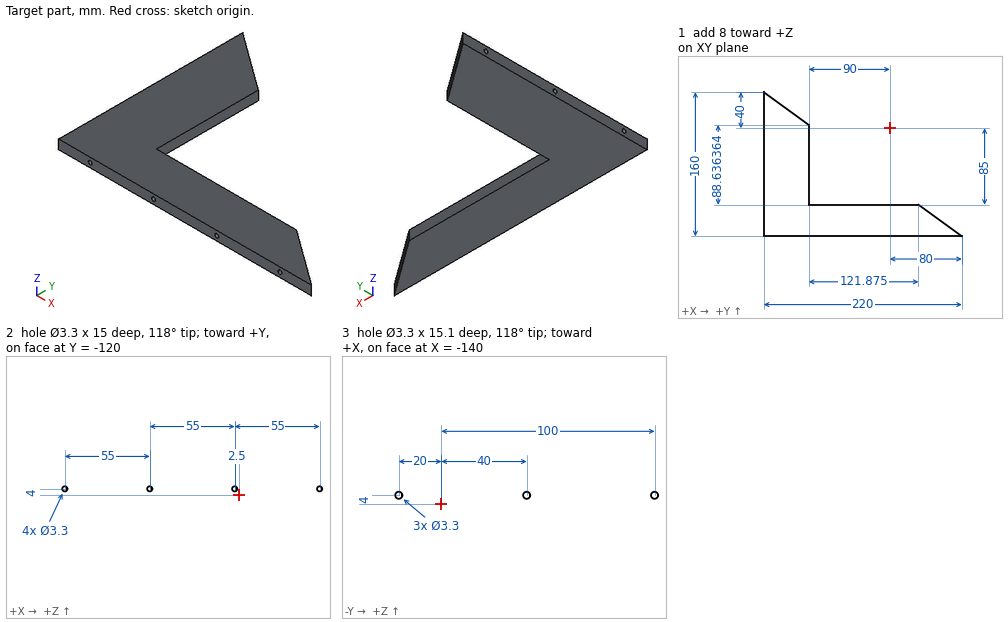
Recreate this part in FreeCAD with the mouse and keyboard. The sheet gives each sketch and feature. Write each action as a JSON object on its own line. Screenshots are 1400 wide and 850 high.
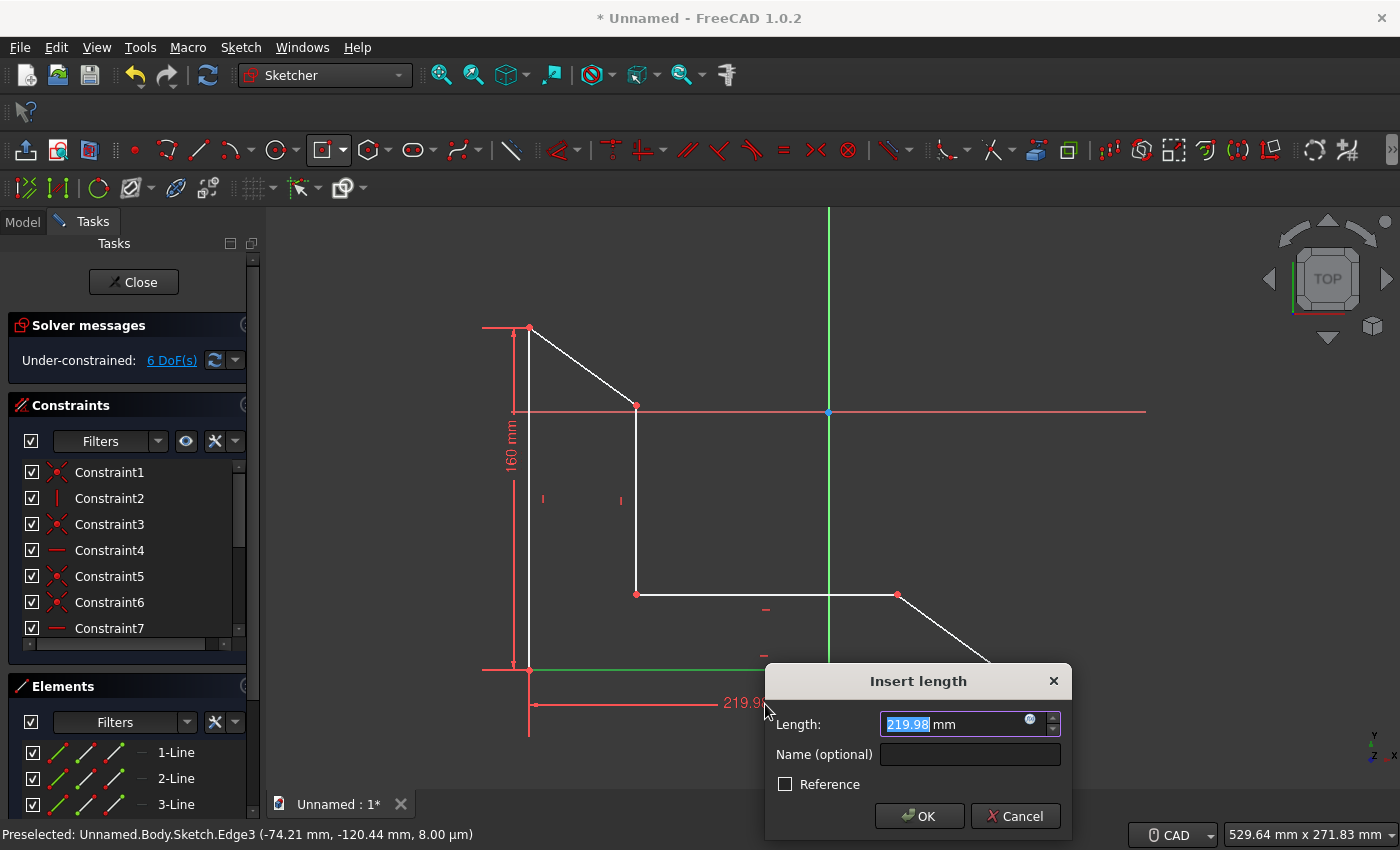
{"action": "type", "text": "220"}
{"action": "key", "text": "Return"}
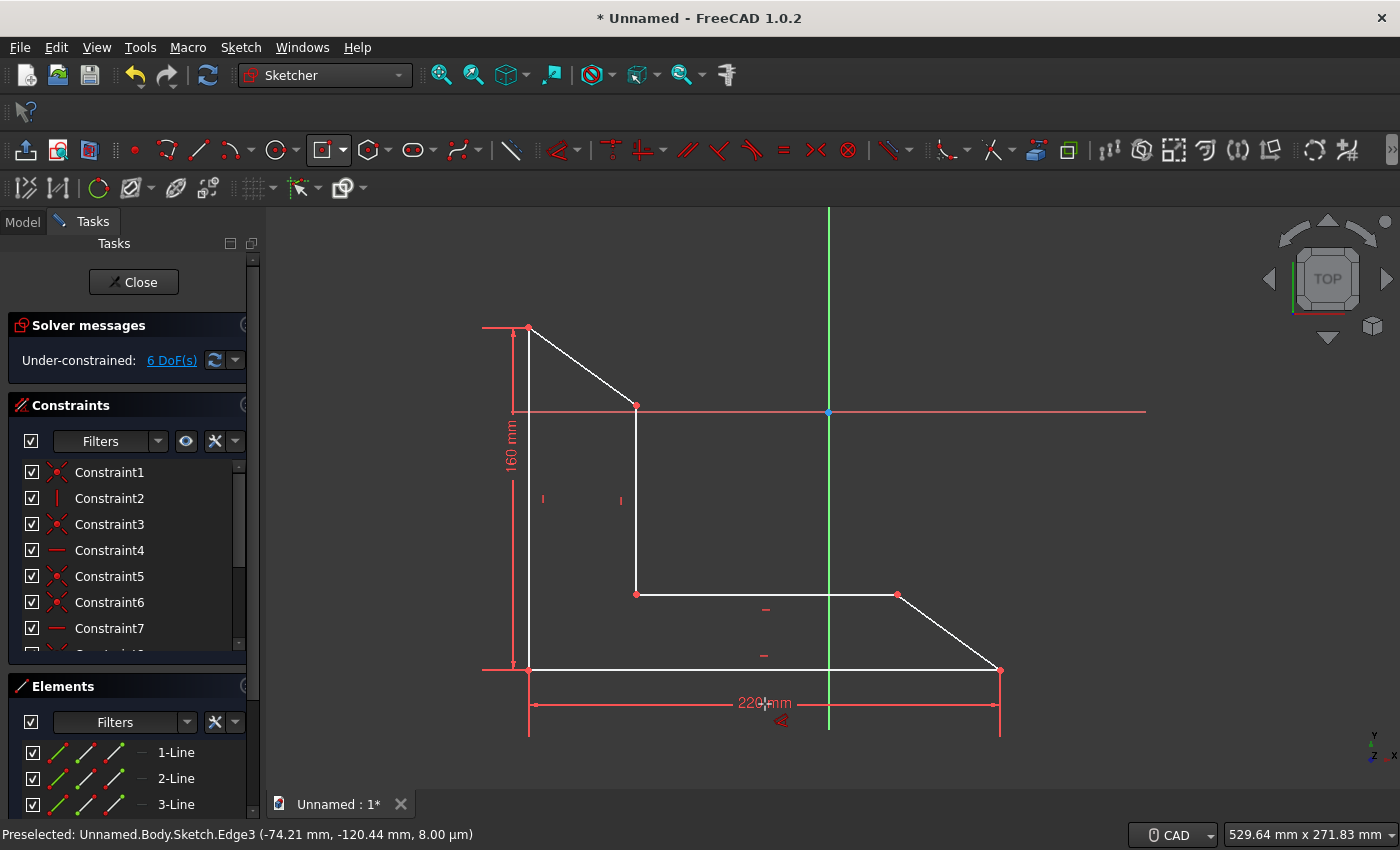
{"action": "left_click", "coordinate": [636, 405]}
{"action": "left_click", "coordinate": [732, 371]}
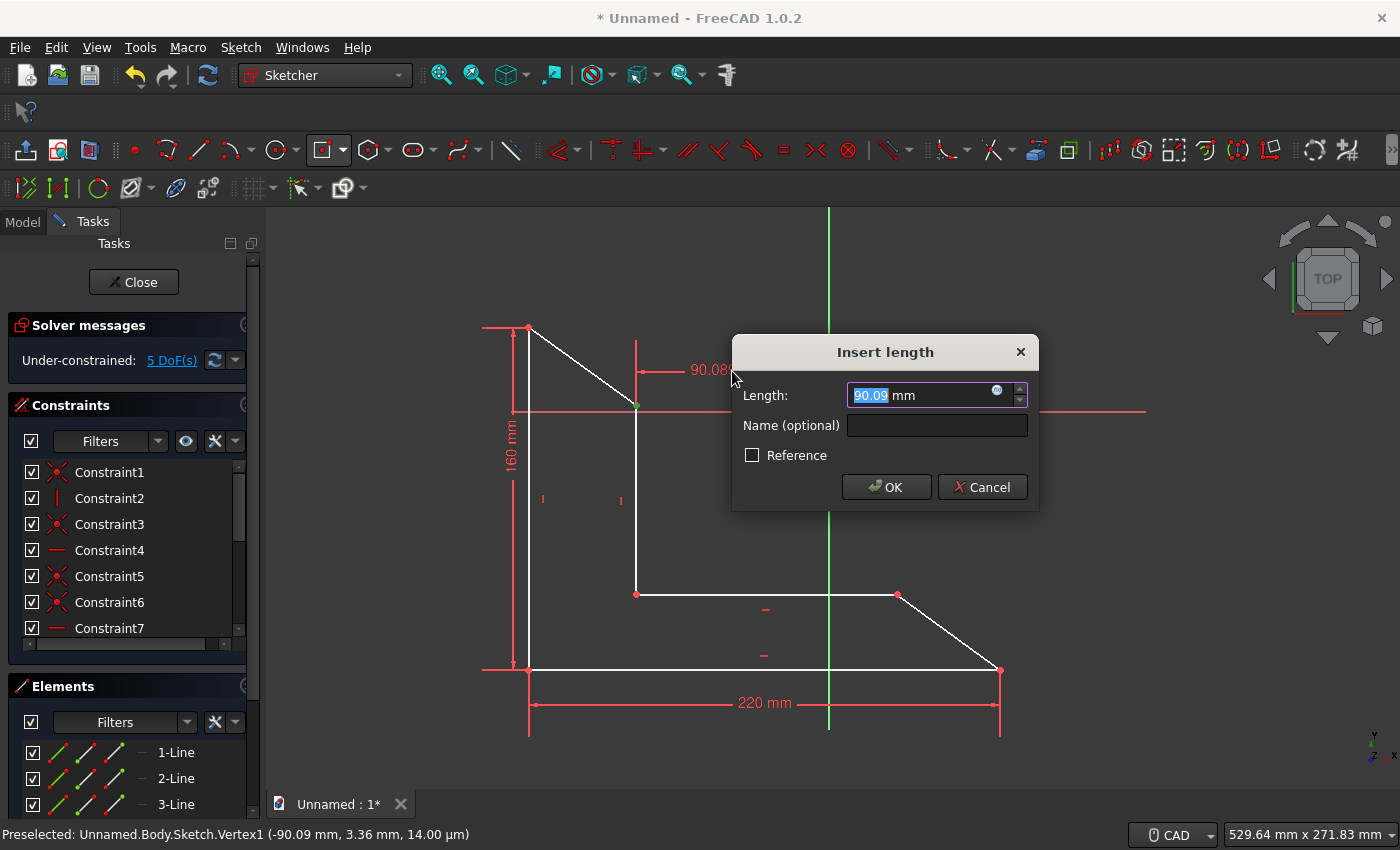
{"action": "type", "text": "90"}
{"action": "key", "text": "Return"}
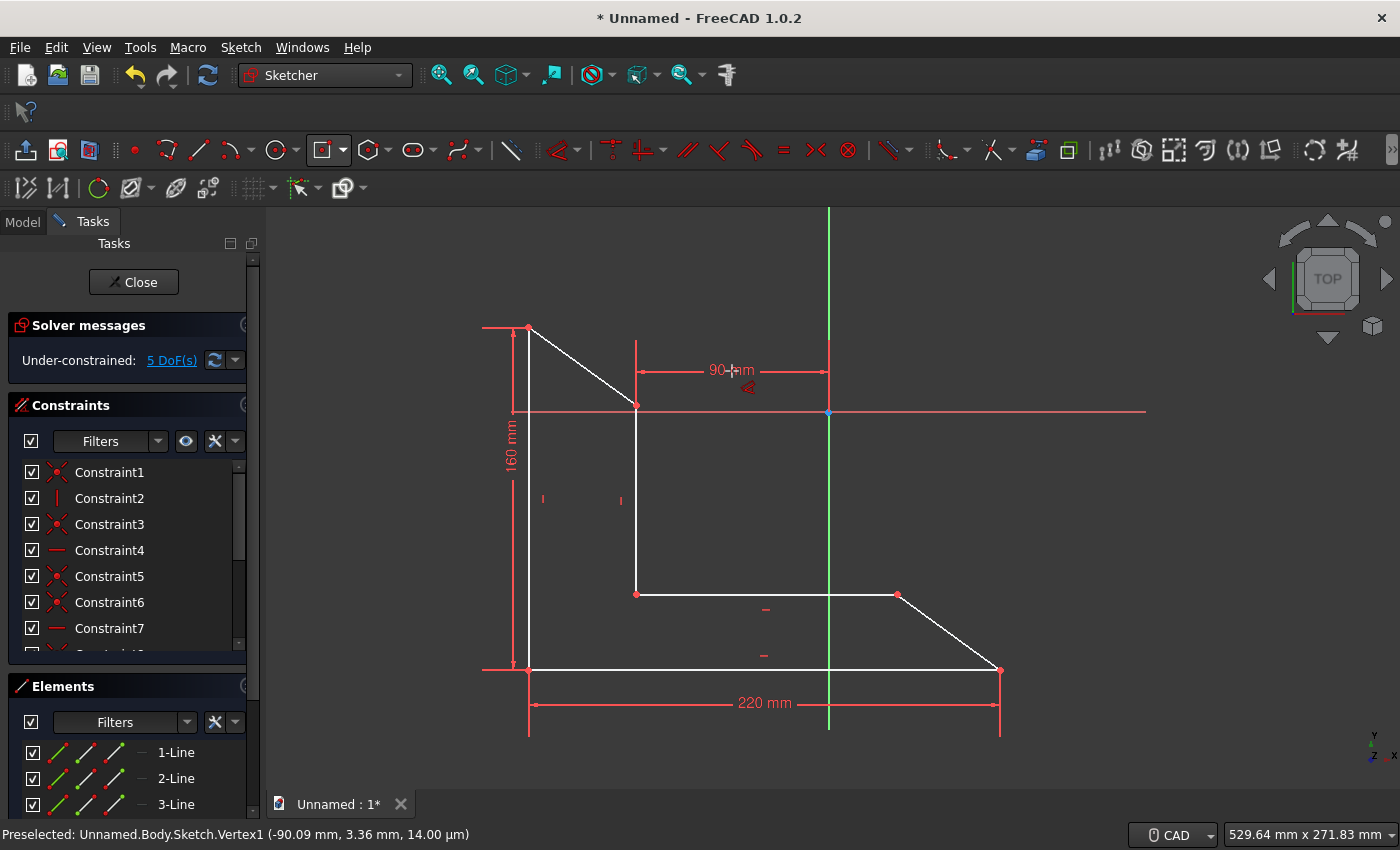
{"action": "left_click", "coordinate": [529, 328]}
{"action": "left_click", "coordinate": [495, 370]}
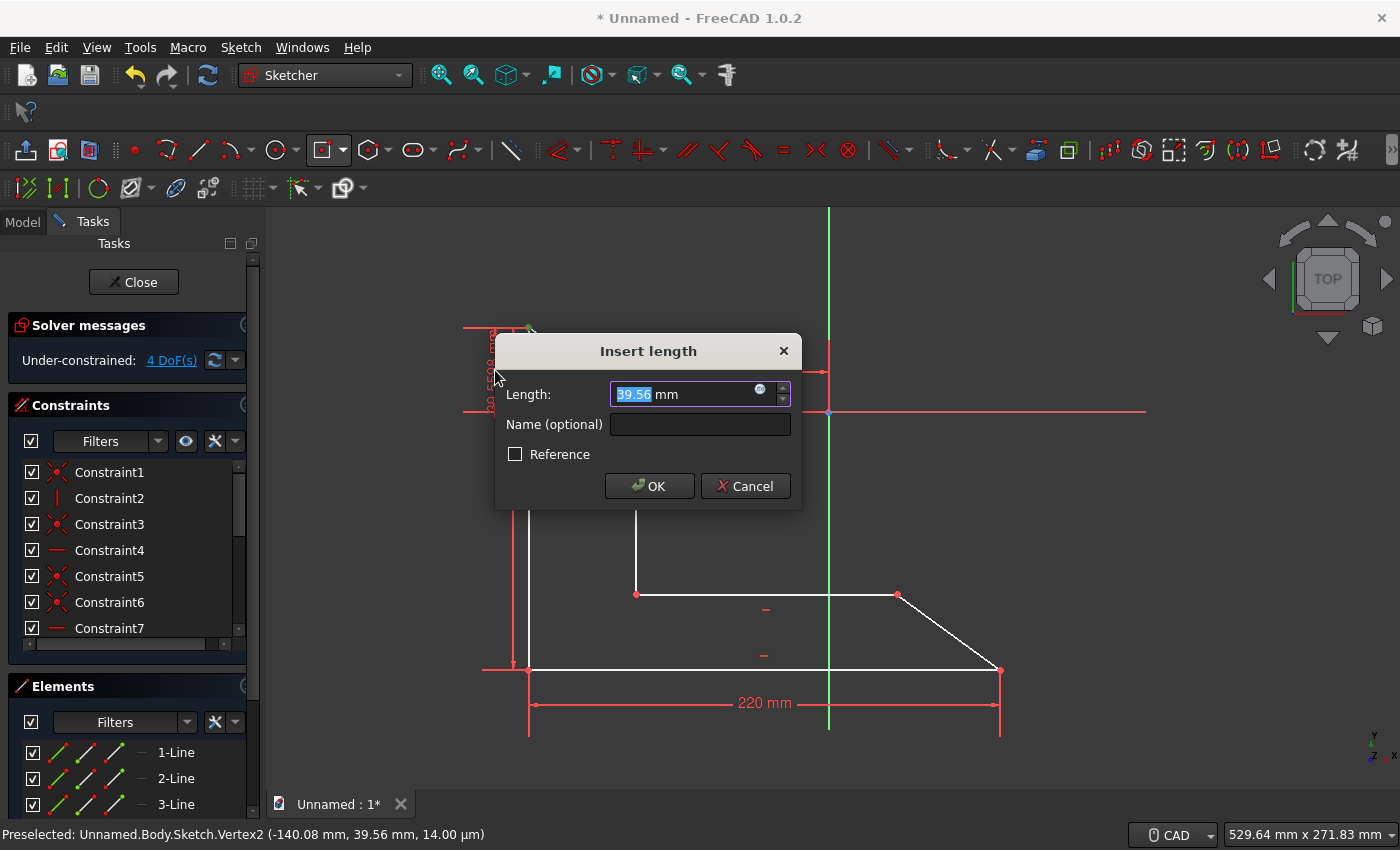
{"action": "type", "text": "40"}
{"action": "key", "text": "Return"}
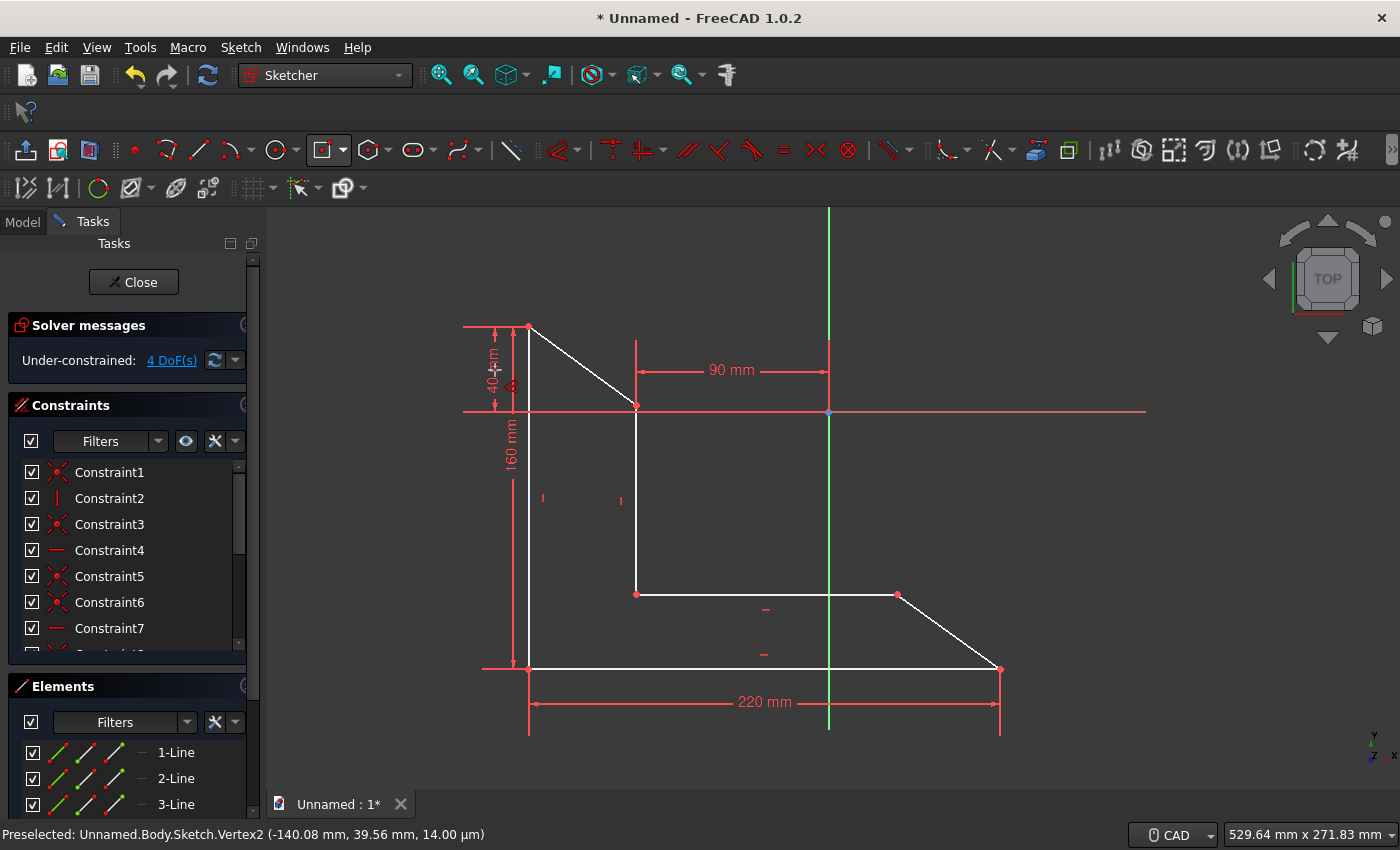
{"action": "left_click", "coordinate": [1000, 669]}
{"action": "left_click", "coordinate": [914, 703]}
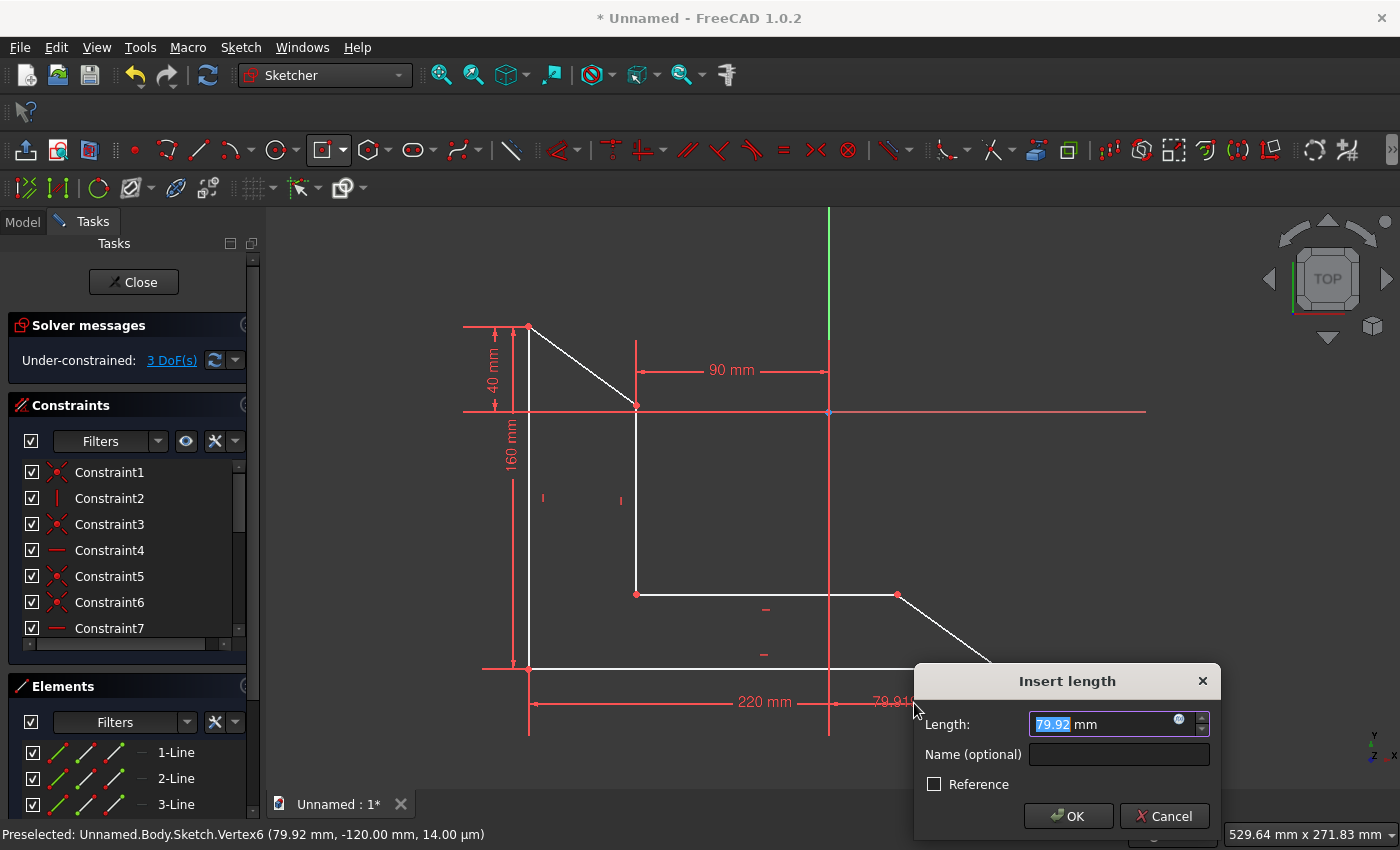
{"action": "type", "text": "80"}
{"action": "key", "text": "Return"}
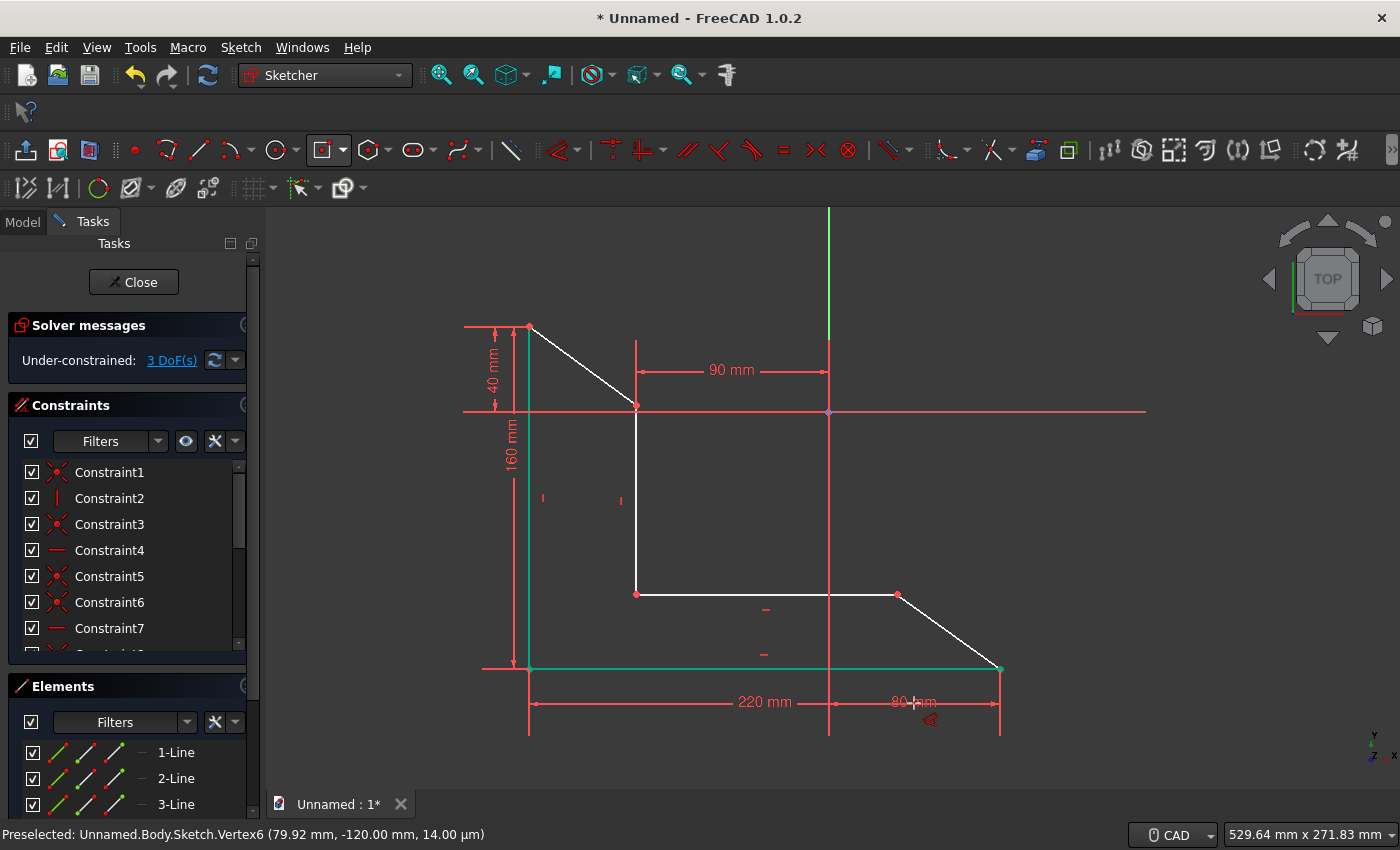
{"action": "left_click", "coordinate": [897, 595]}
{"action": "left_click", "coordinate": [931, 504]}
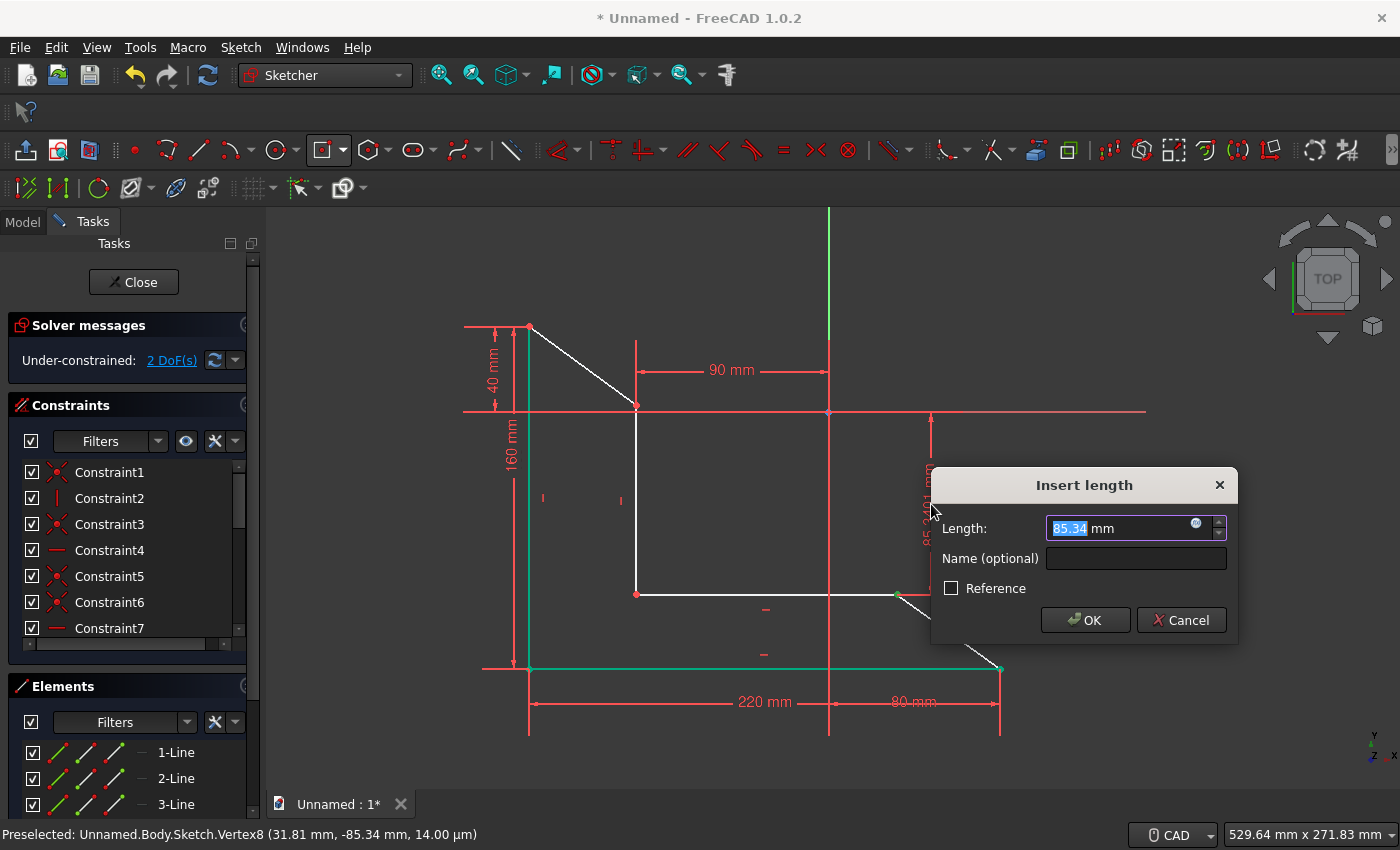
{"action": "type", "text": "85"}
{"action": "key", "text": "Return"}